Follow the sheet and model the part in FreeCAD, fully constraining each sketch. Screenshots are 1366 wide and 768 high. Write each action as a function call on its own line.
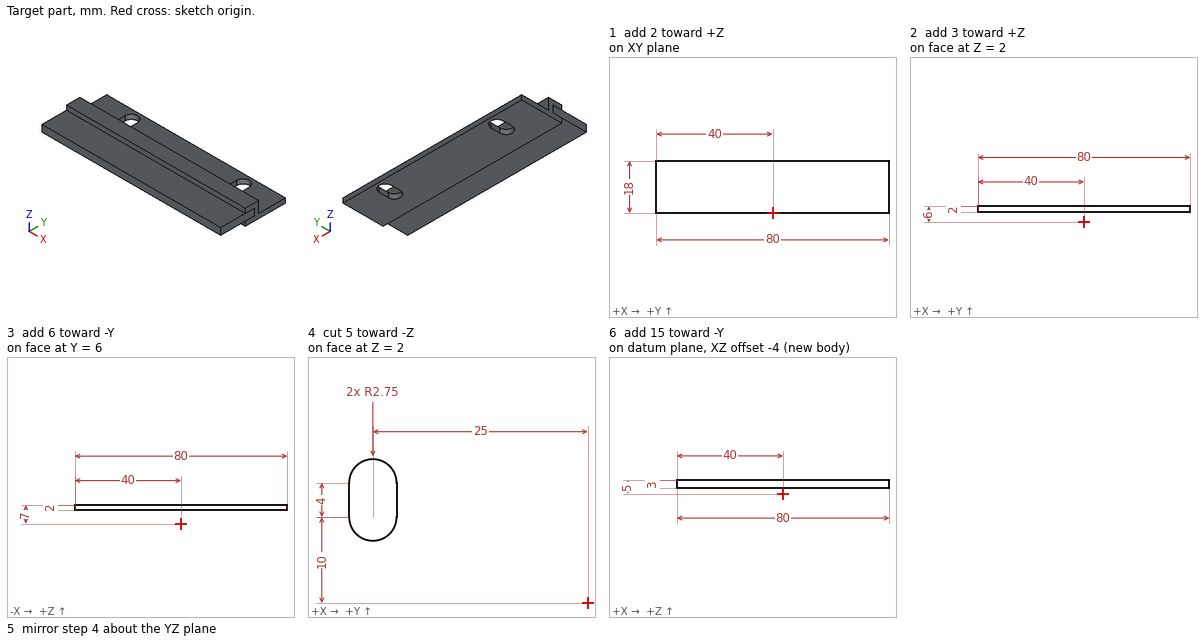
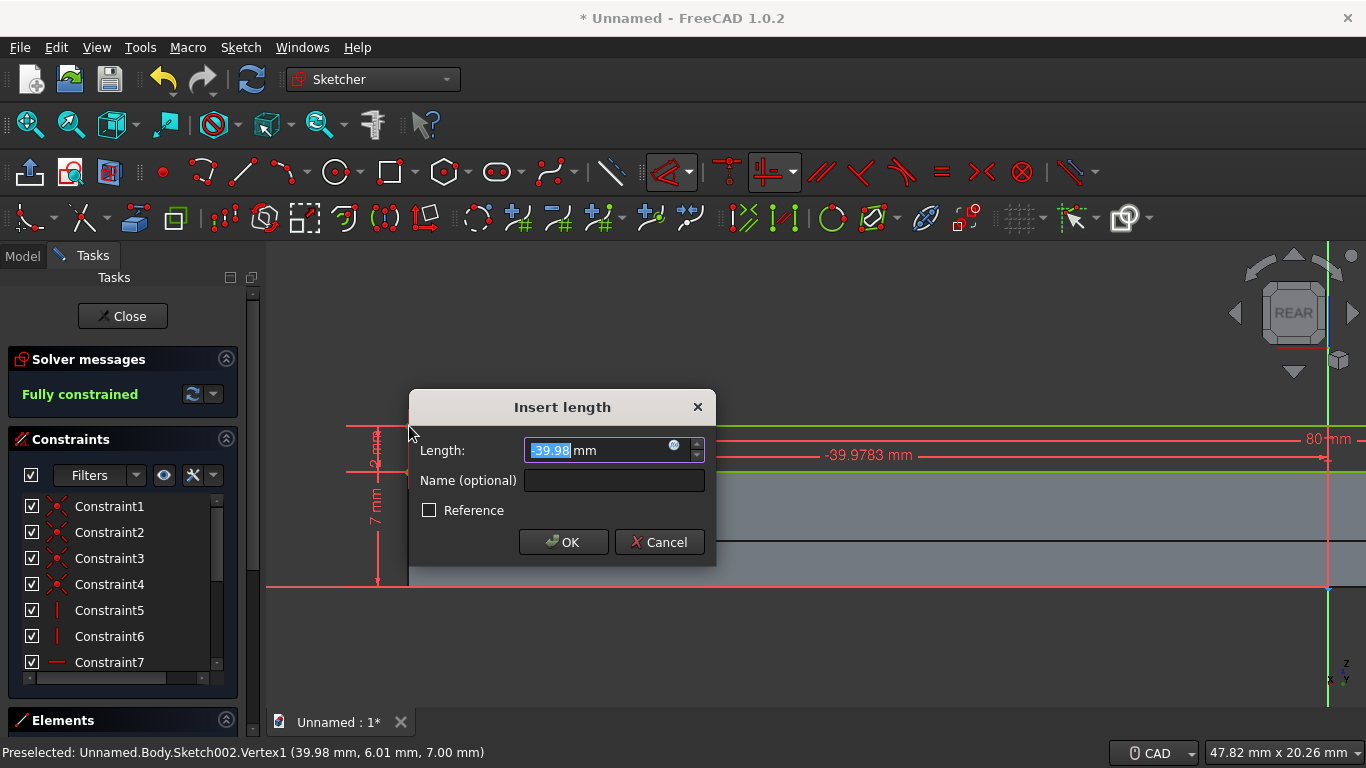
text(-40)
key(Return)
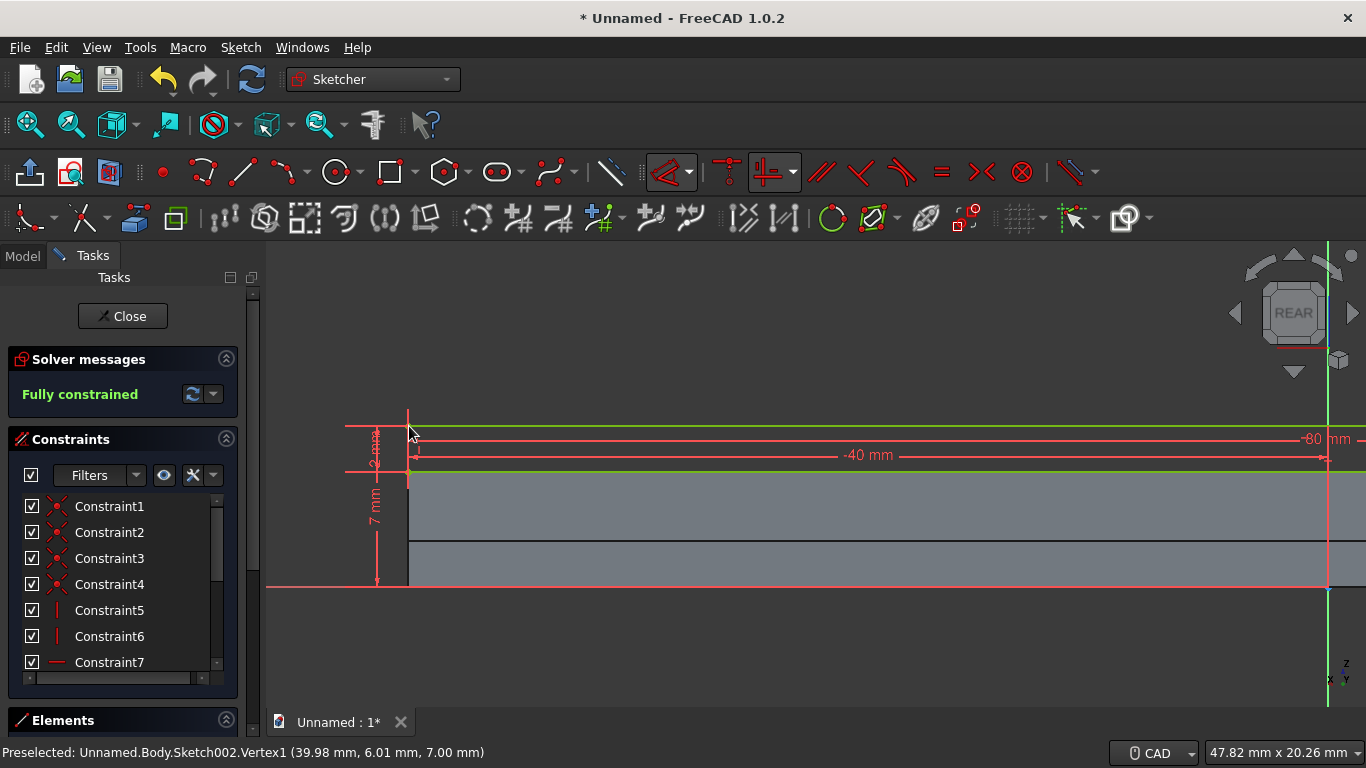
click(123, 316)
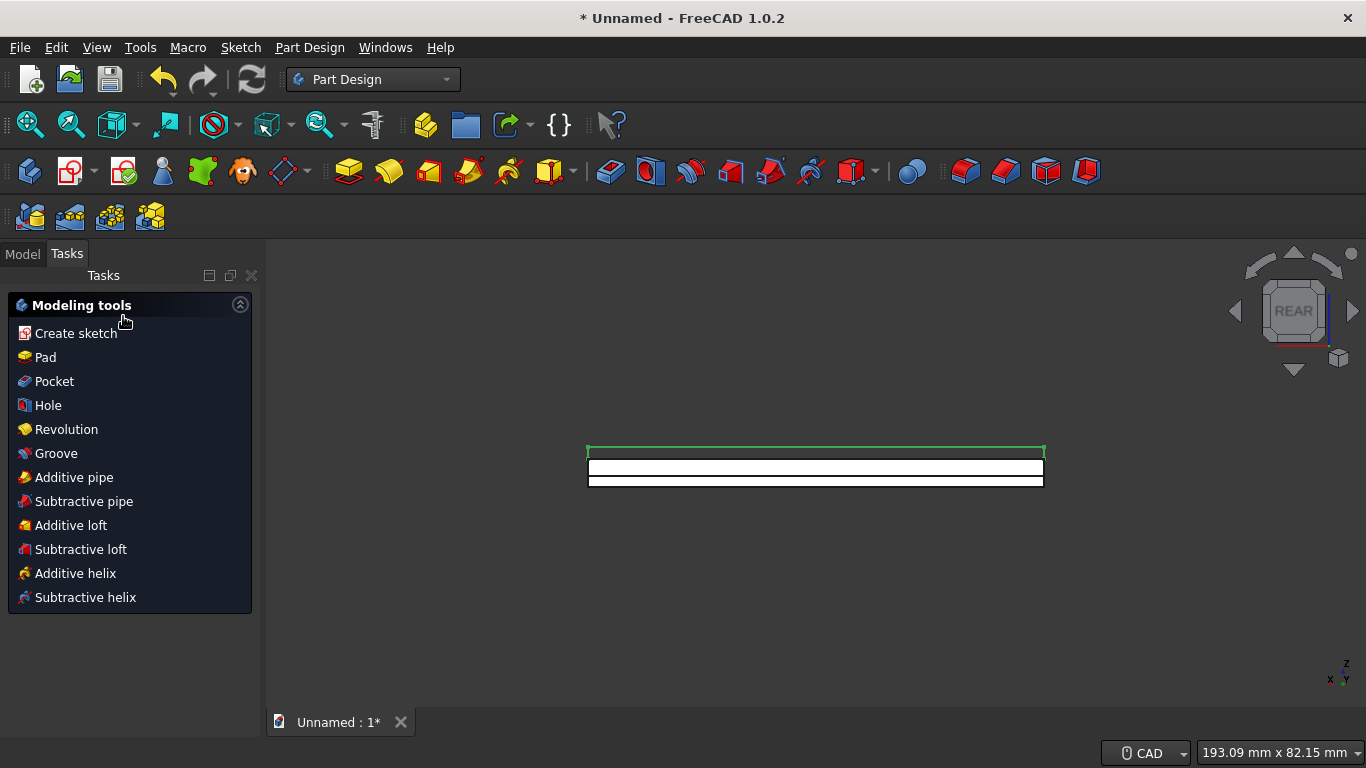
click(350, 172)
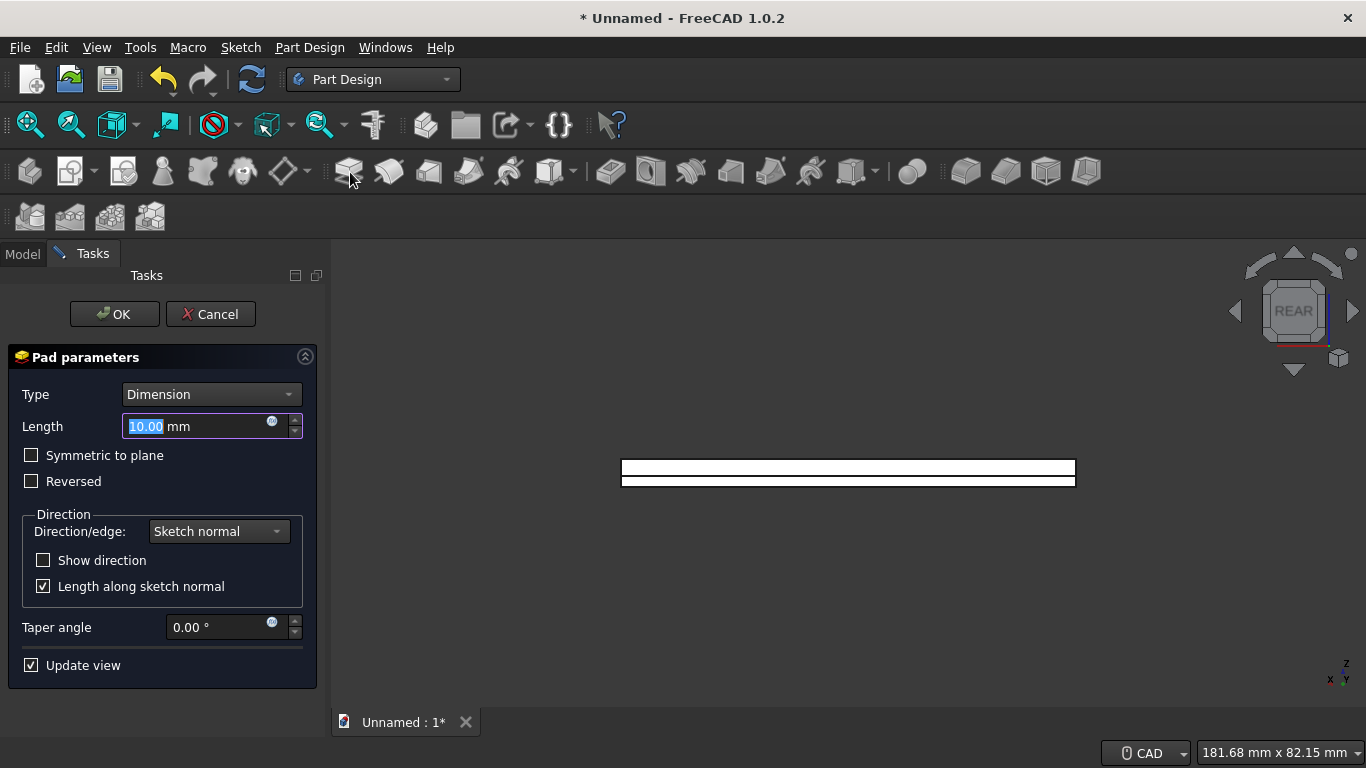
text(6)
key(Tab)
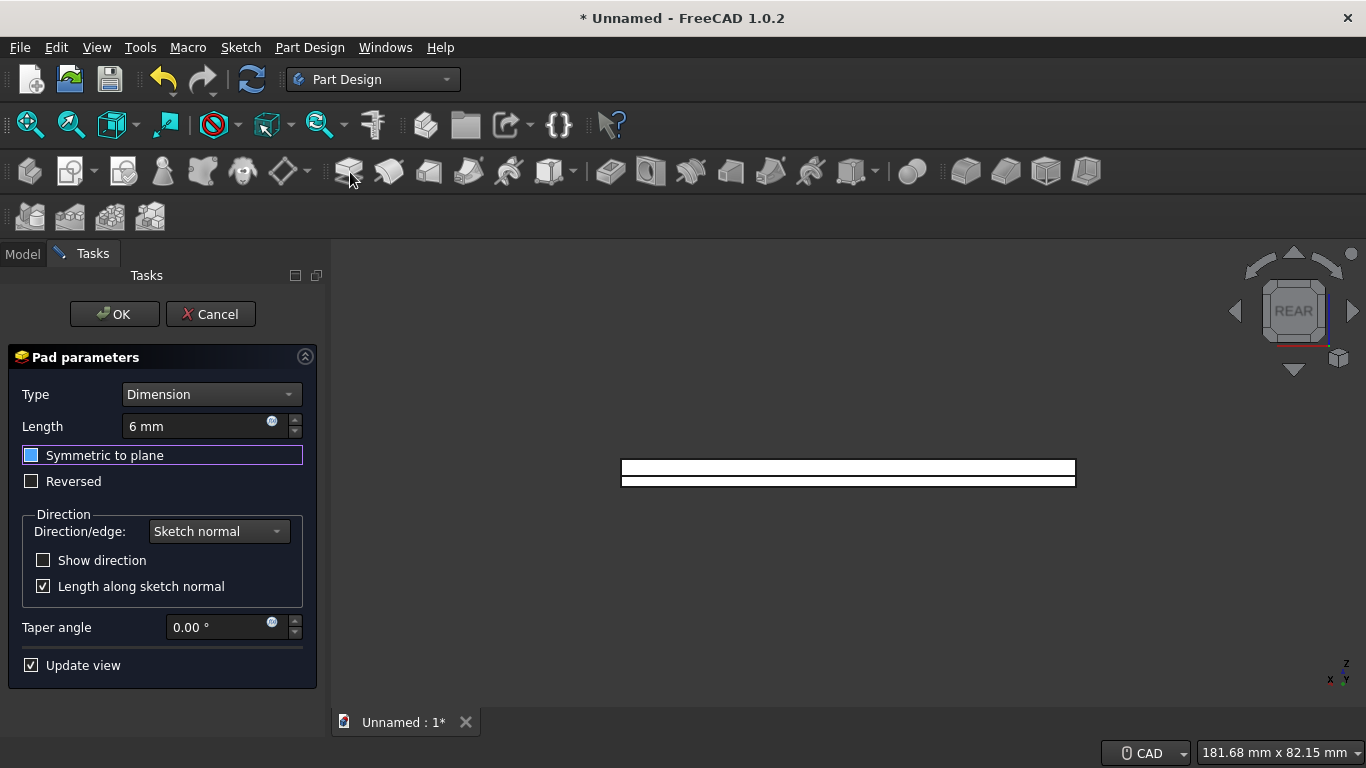
click(30, 481)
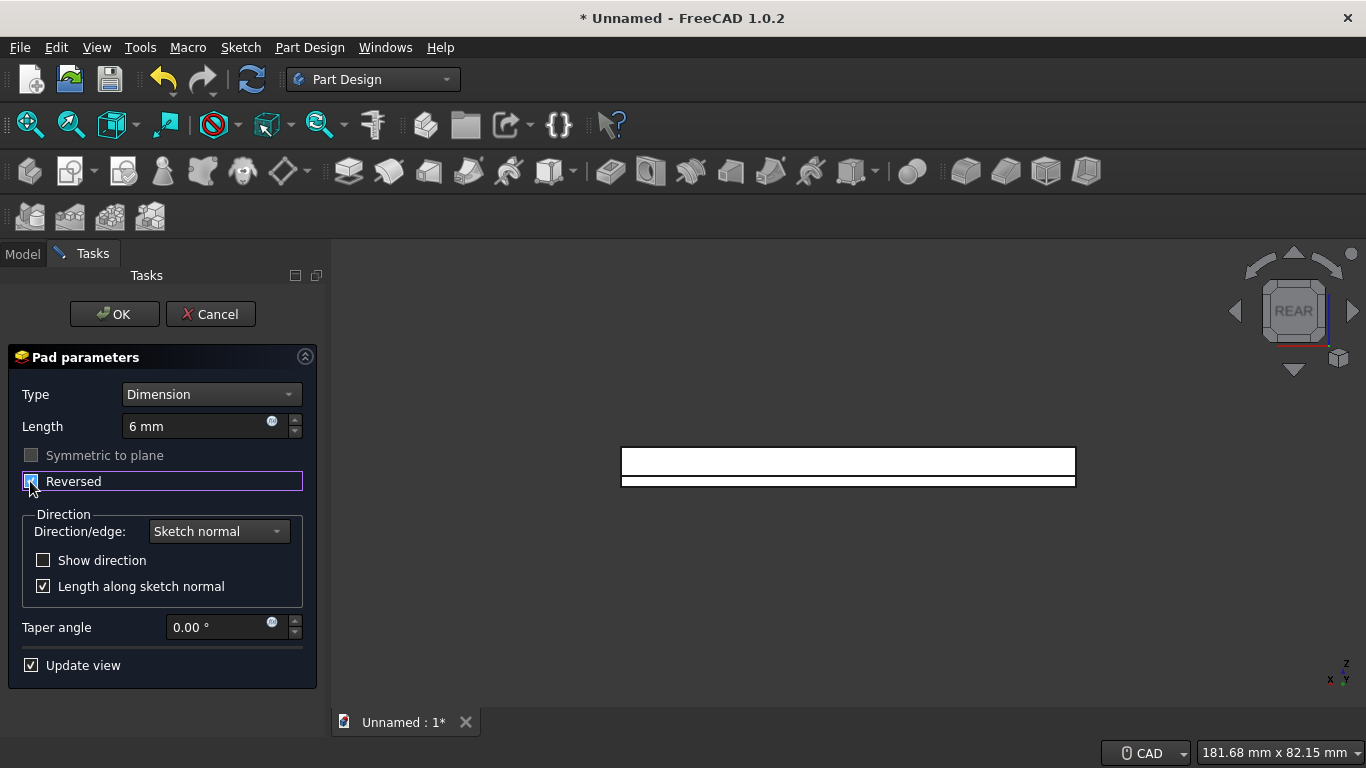
click(115, 314)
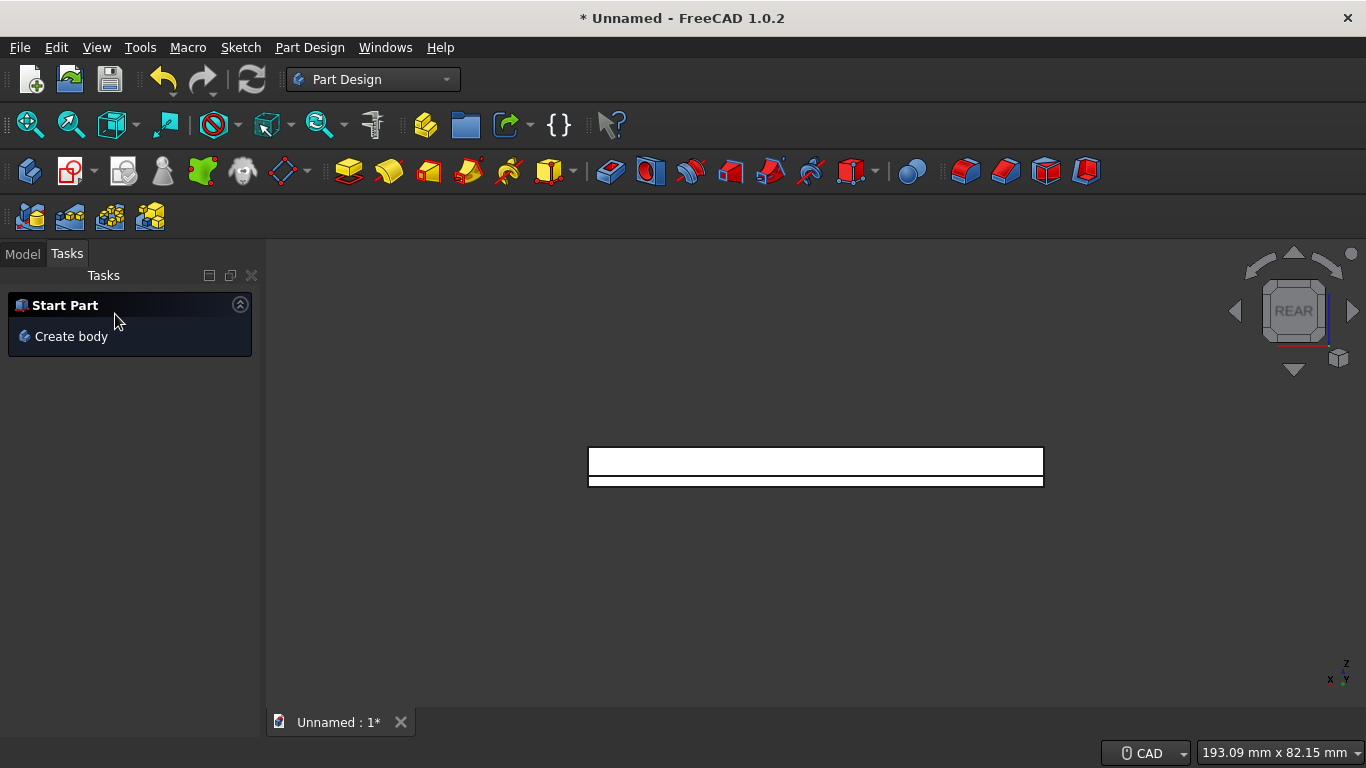
key(v)
key(f)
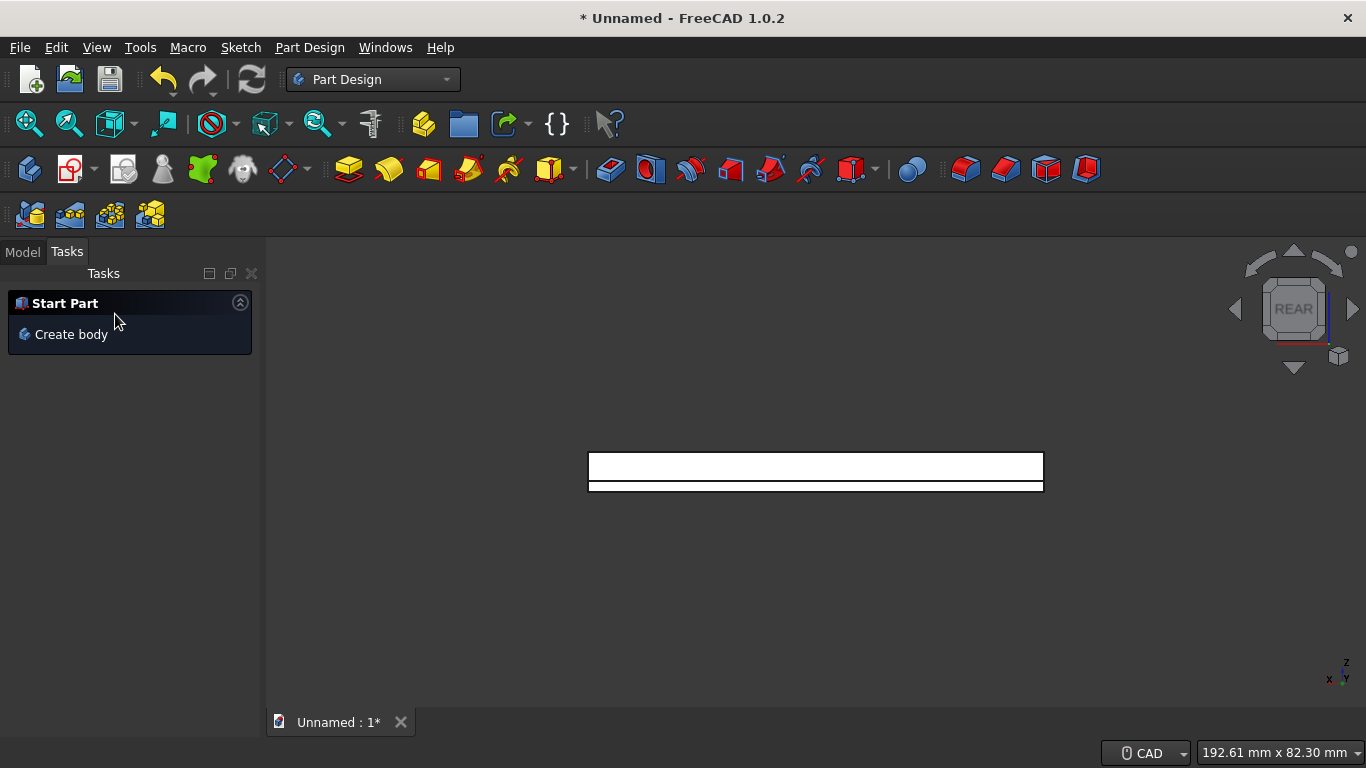
key(0)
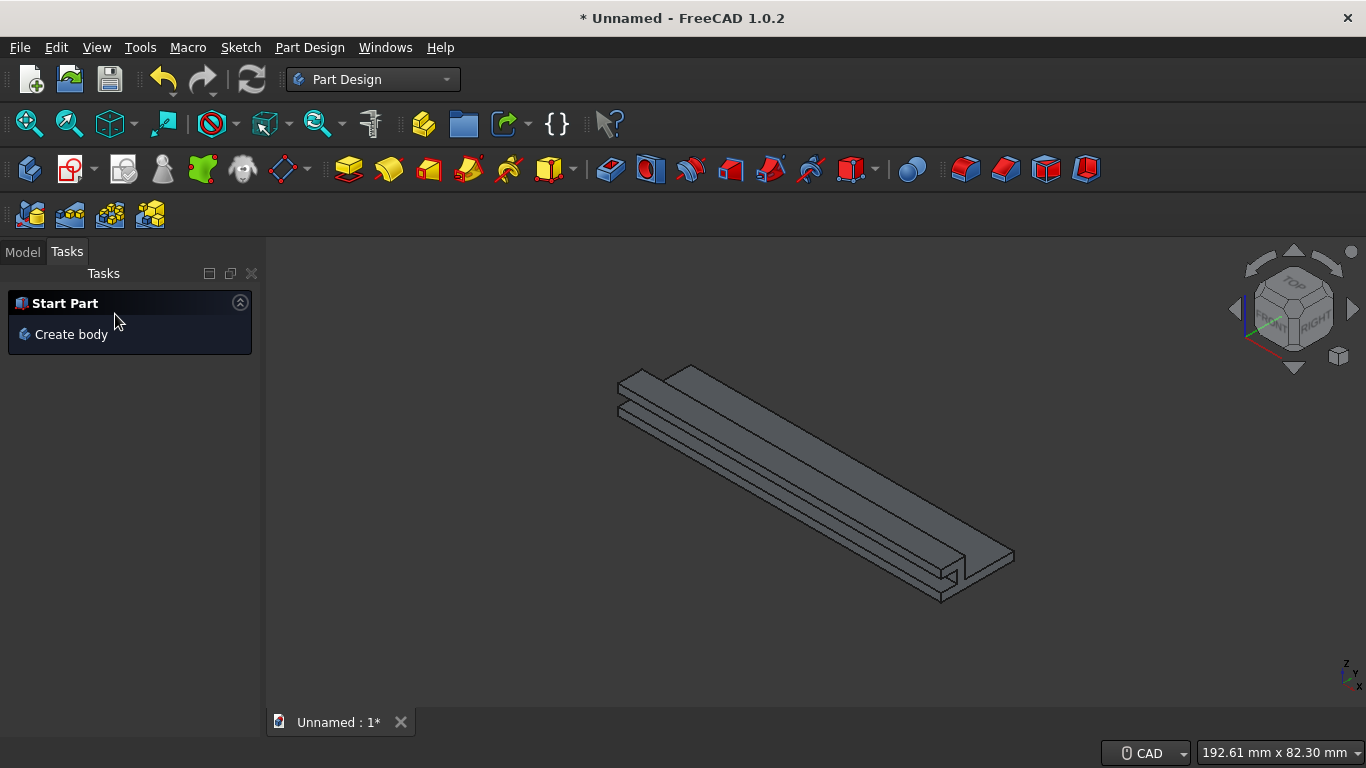
click(973, 547)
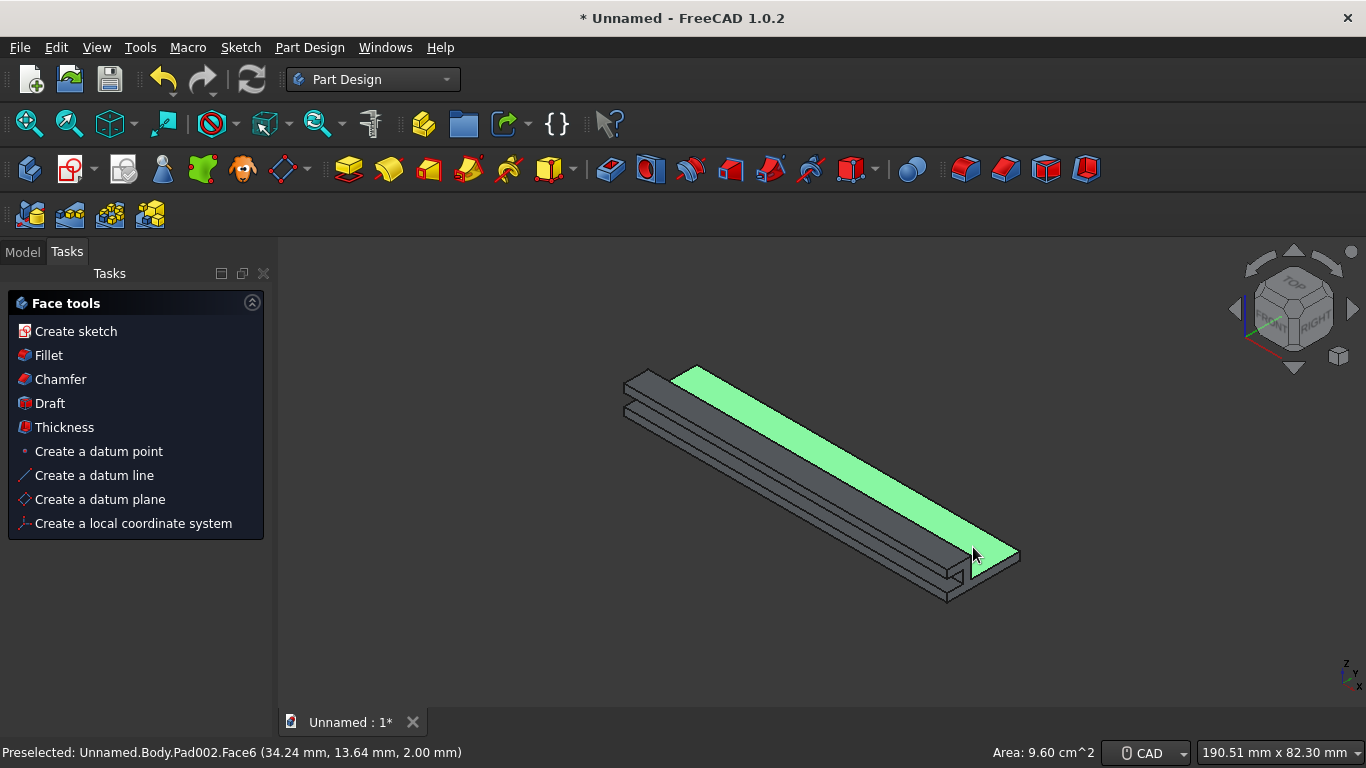
click(70, 170)